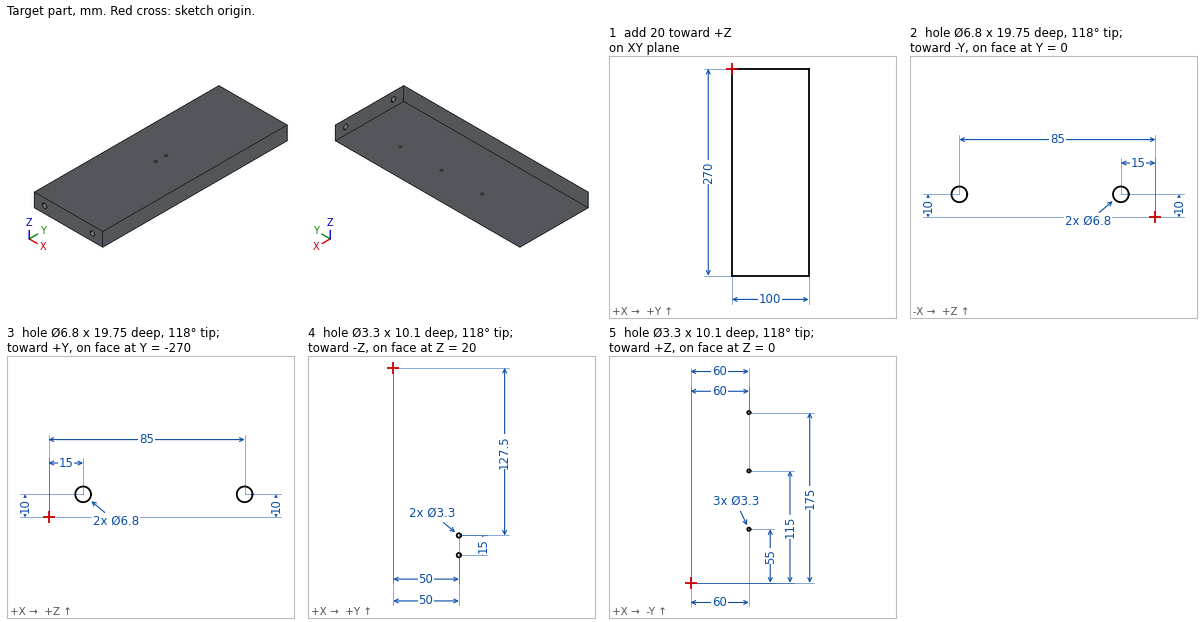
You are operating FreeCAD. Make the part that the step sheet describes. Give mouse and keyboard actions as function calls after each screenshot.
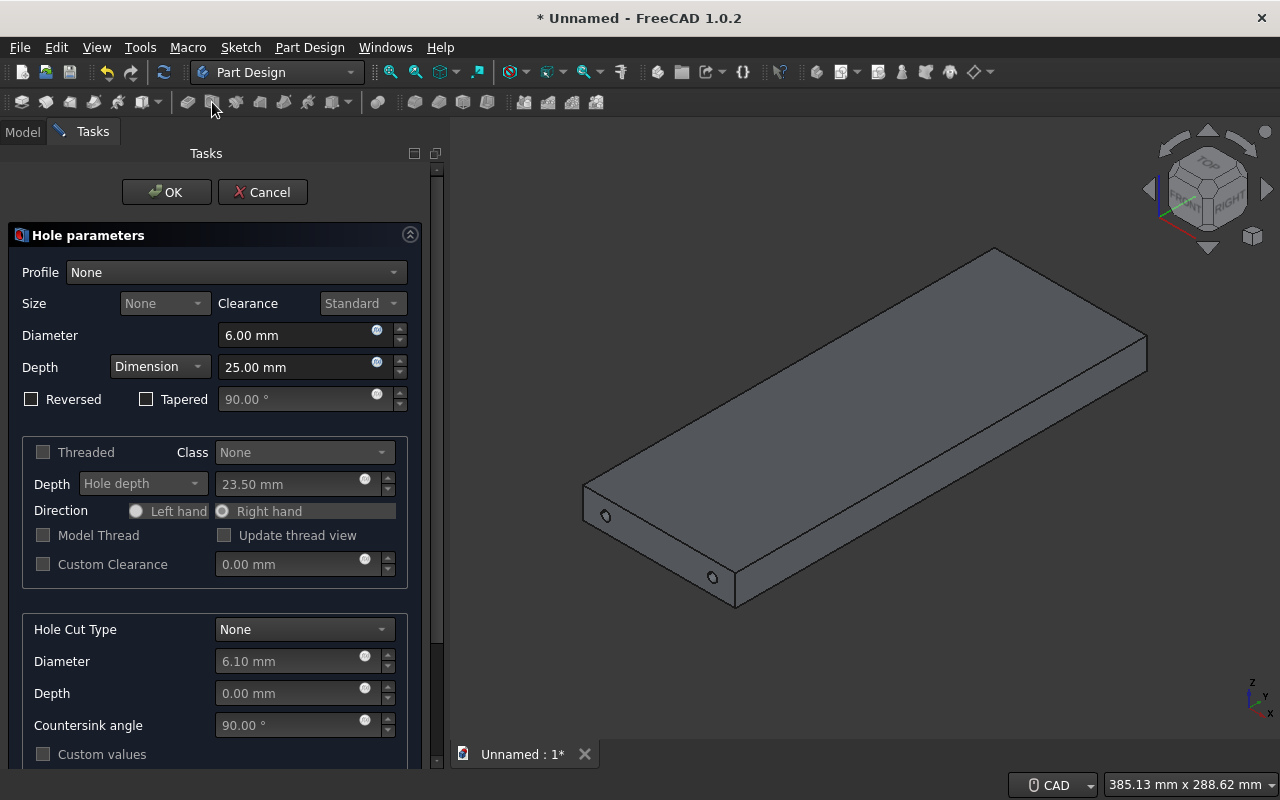
triple_click(305, 335)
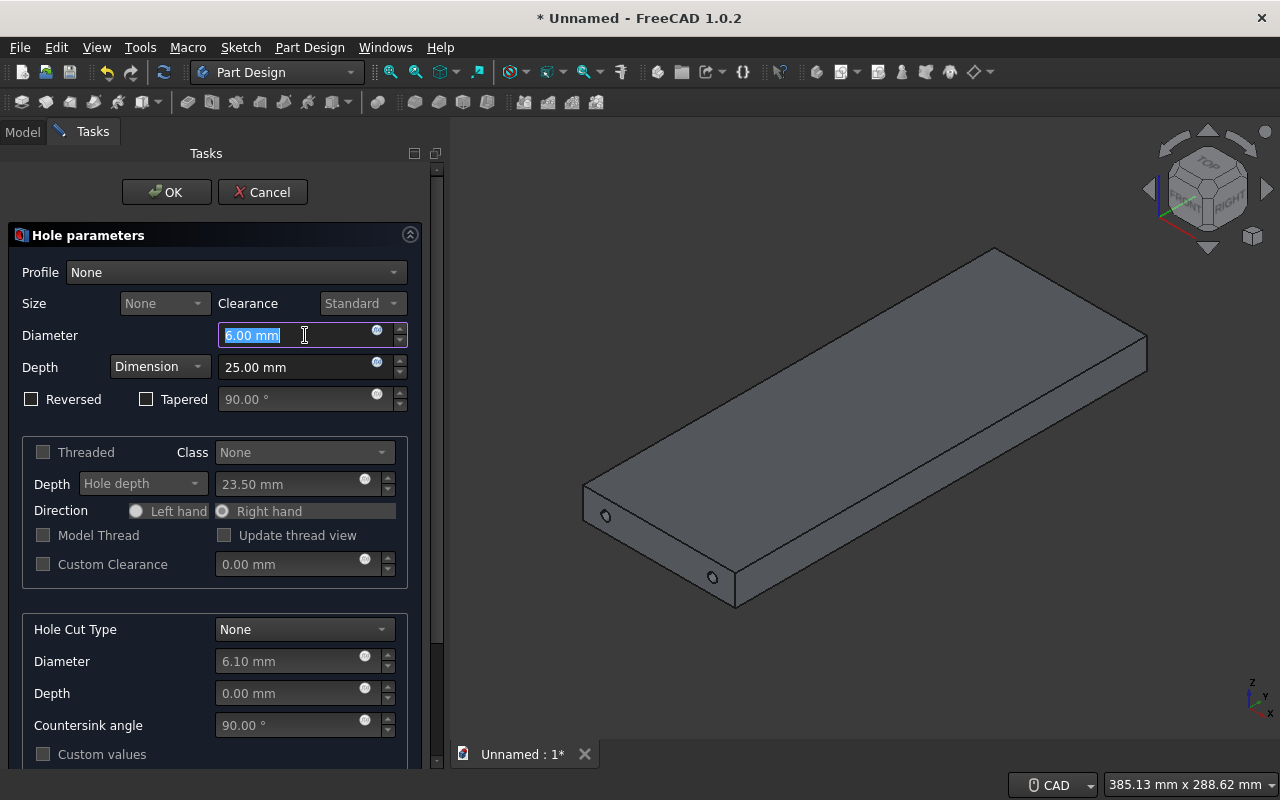
text(6.8)
key(Tab)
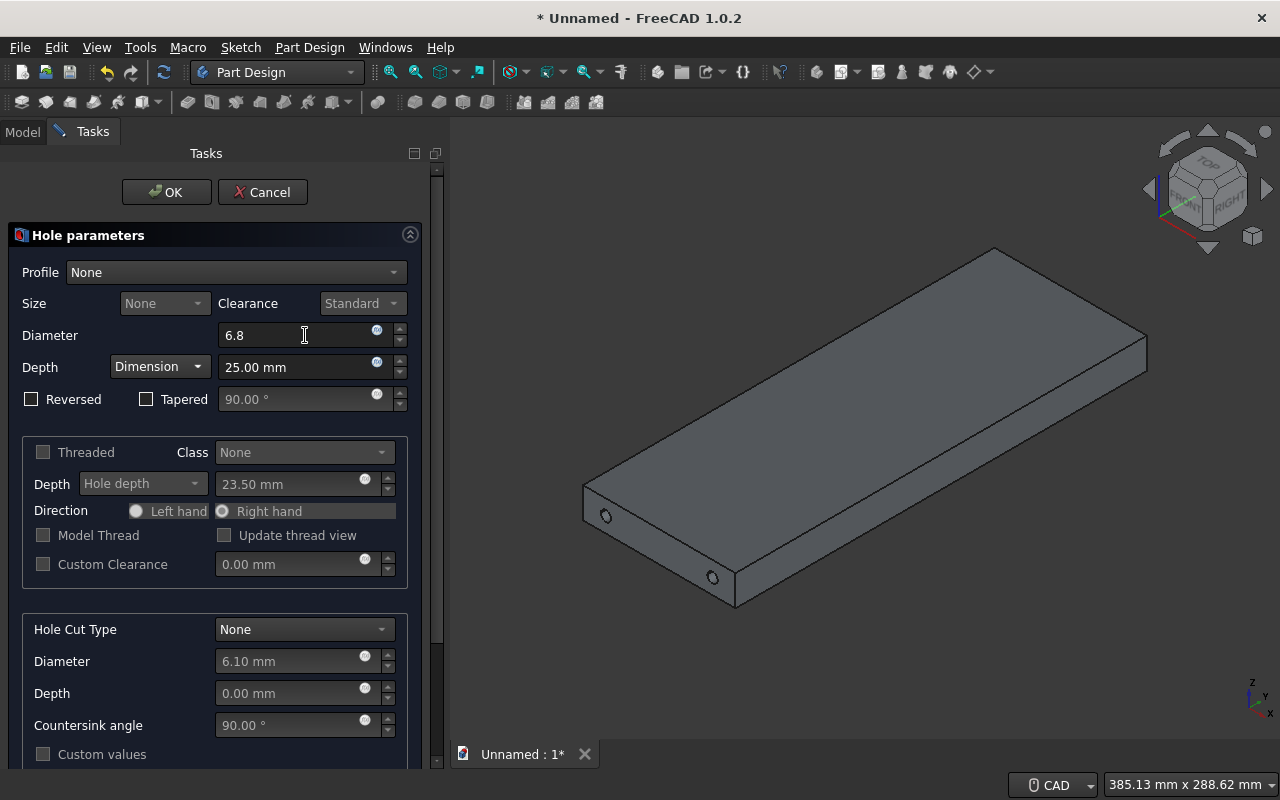
triple_click(305, 367)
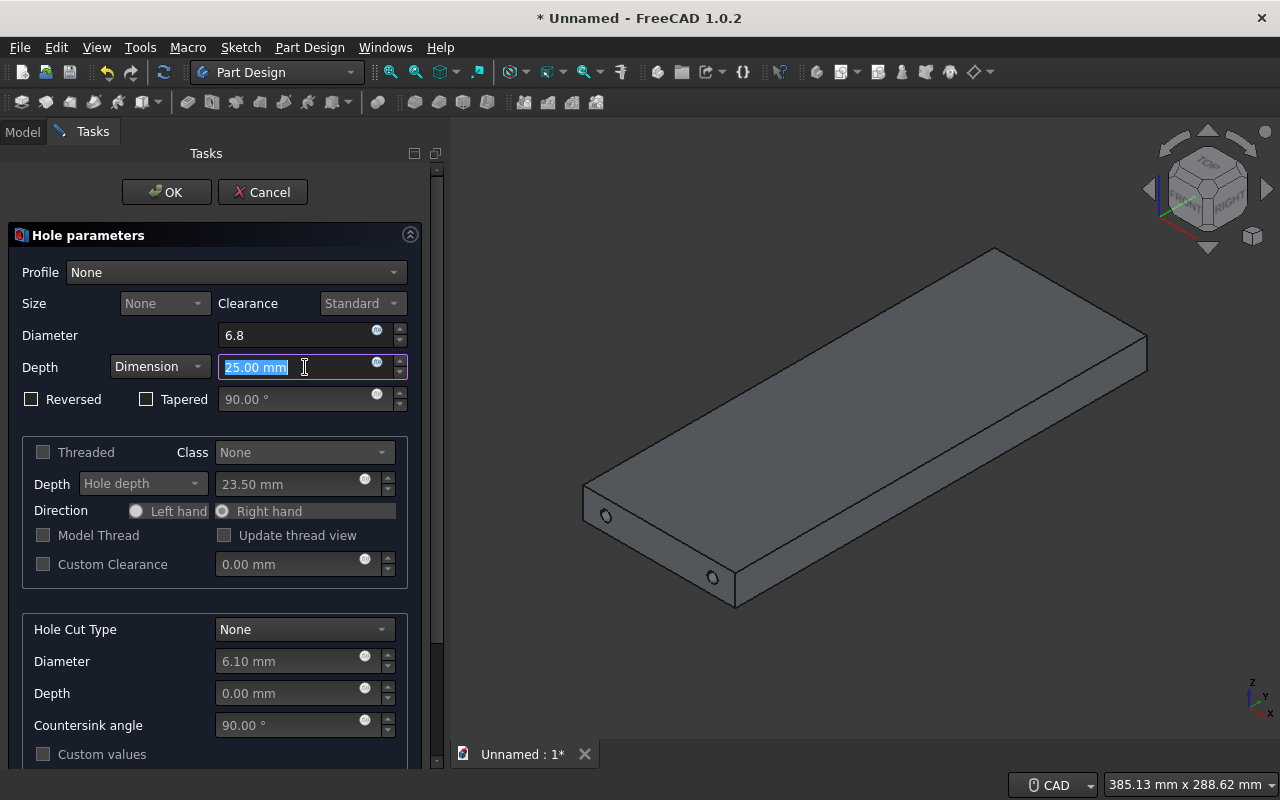
text(19.75)
key(Tab)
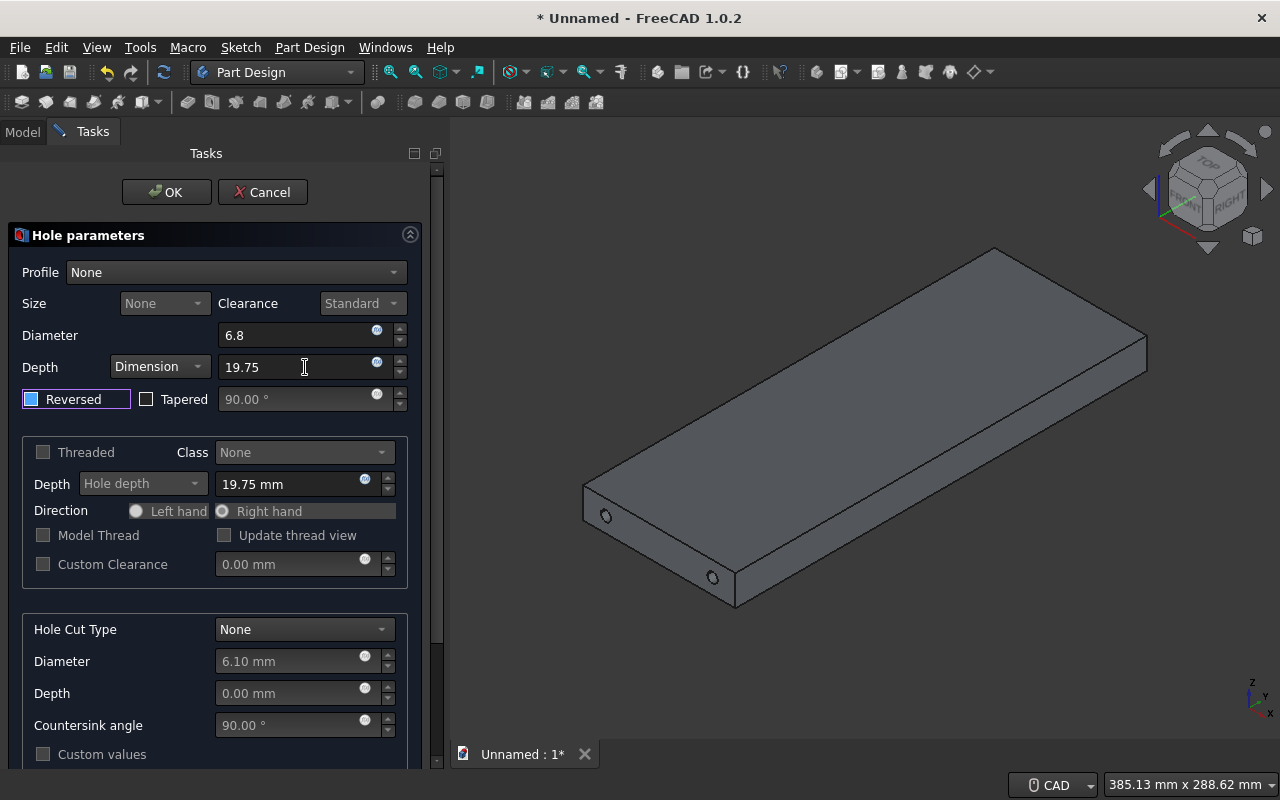
click(167, 192)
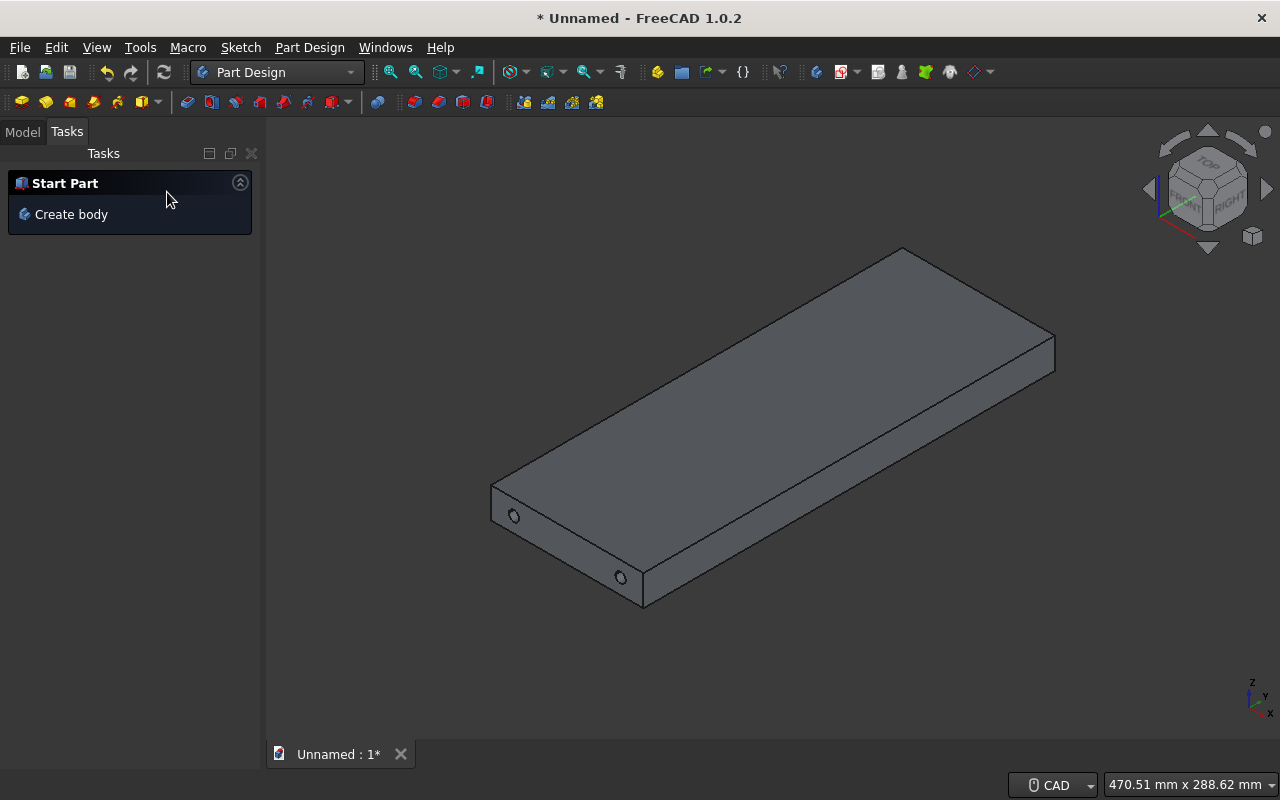
click(891, 342)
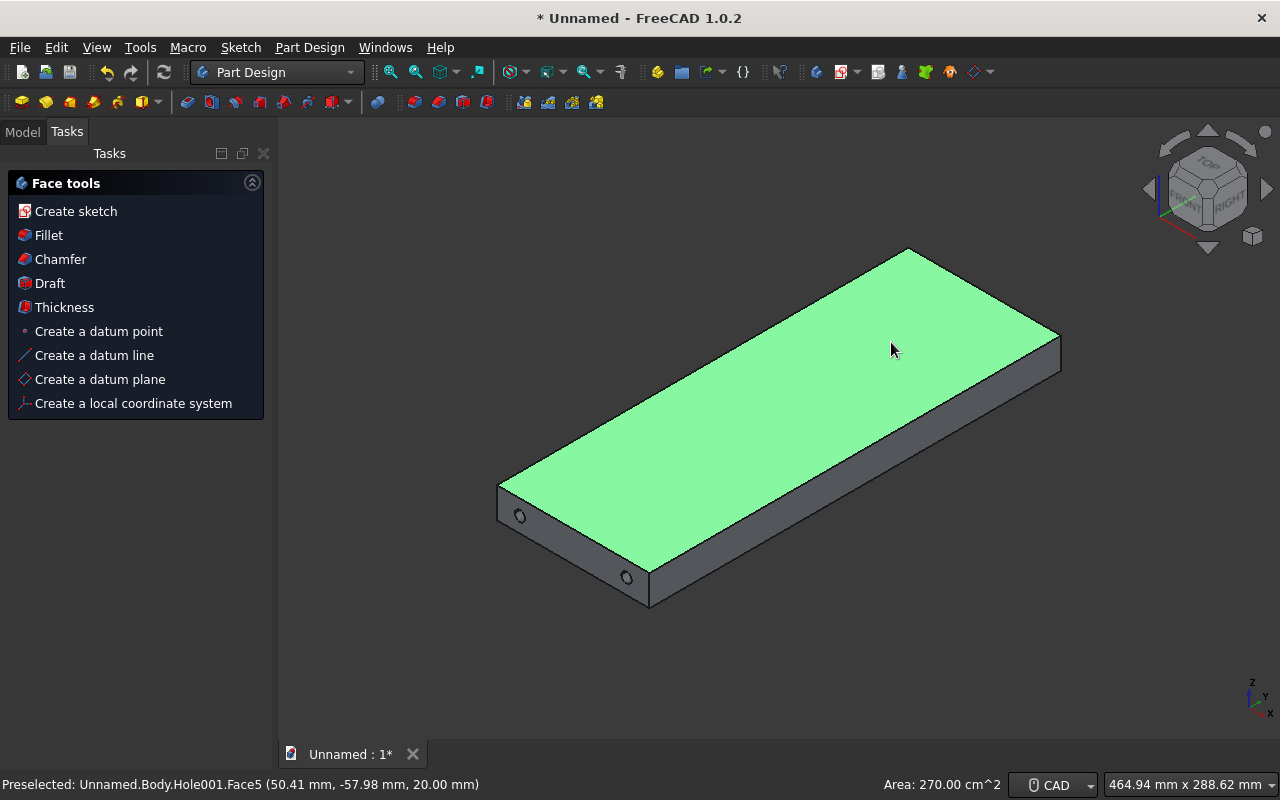
click(842, 72)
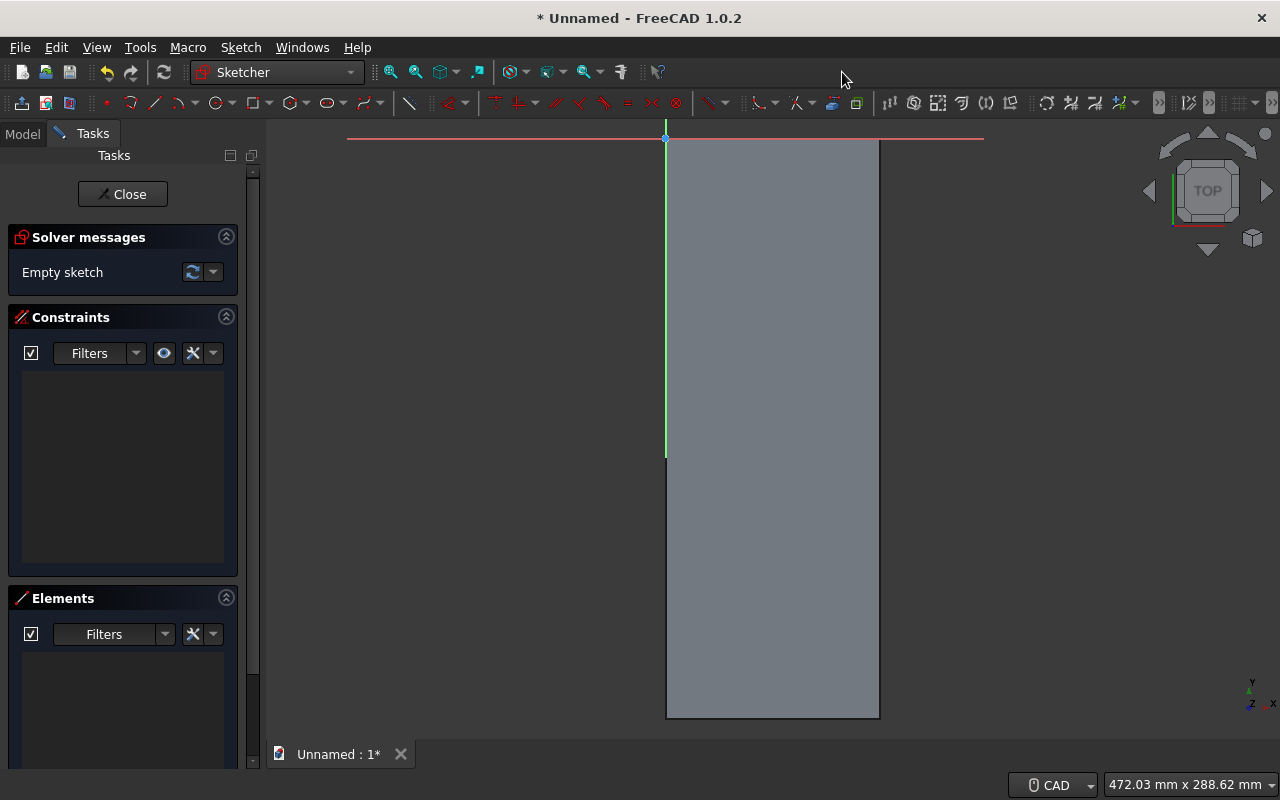
scroll(780, 429, up, 12)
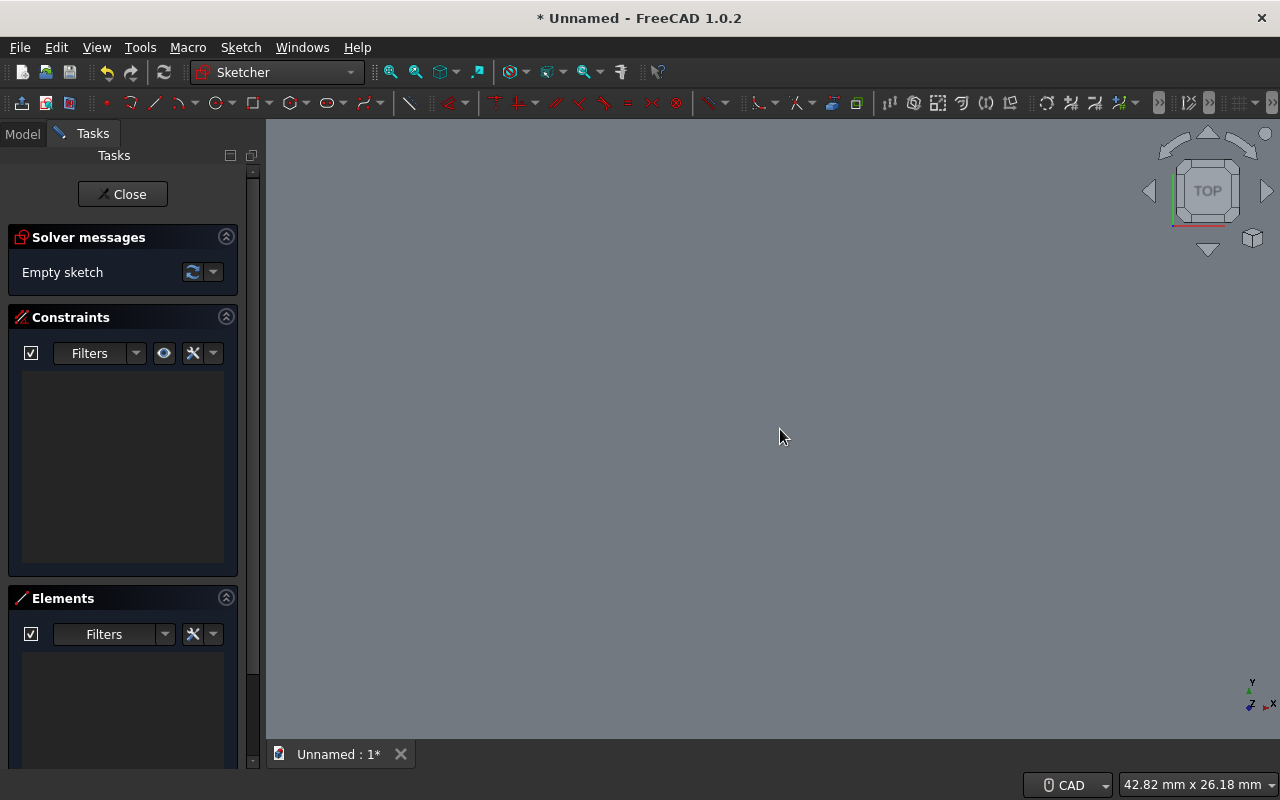
key(g)
key(c)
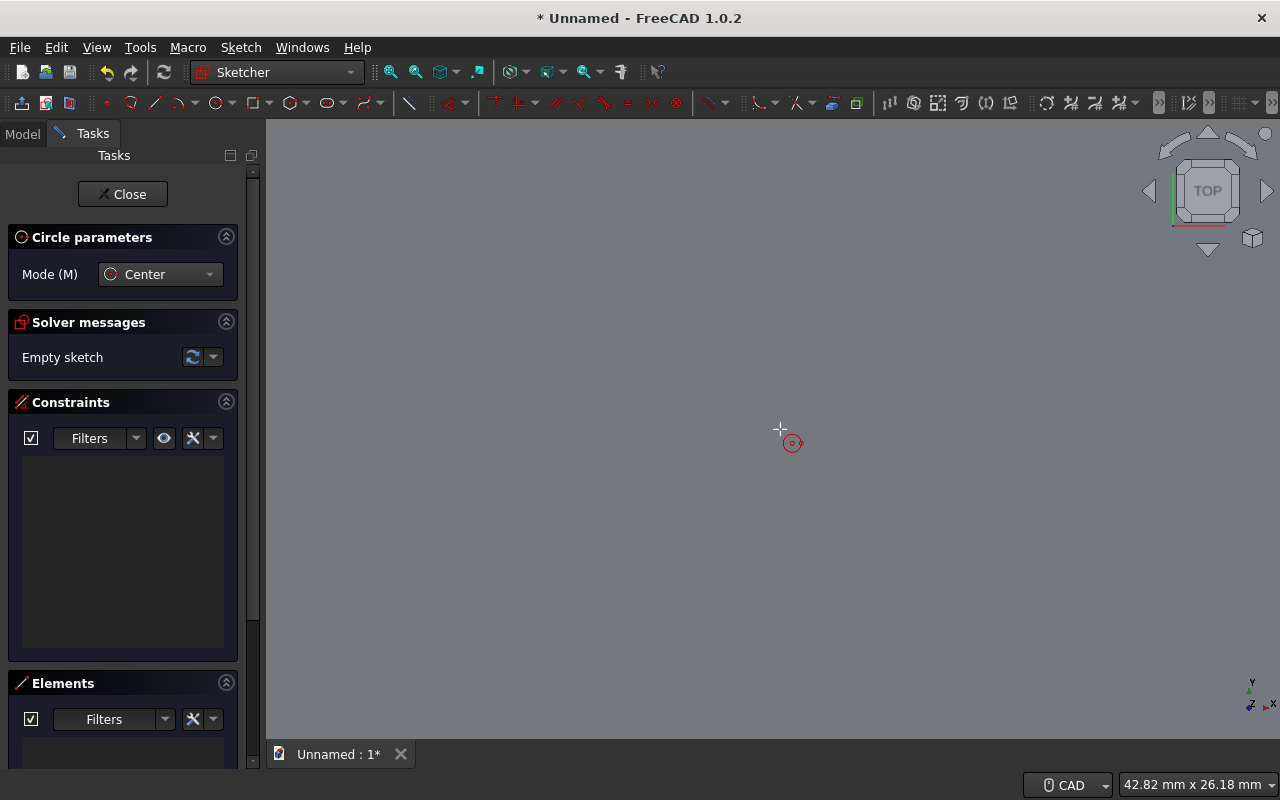
click(698, 246)
click(725, 219)